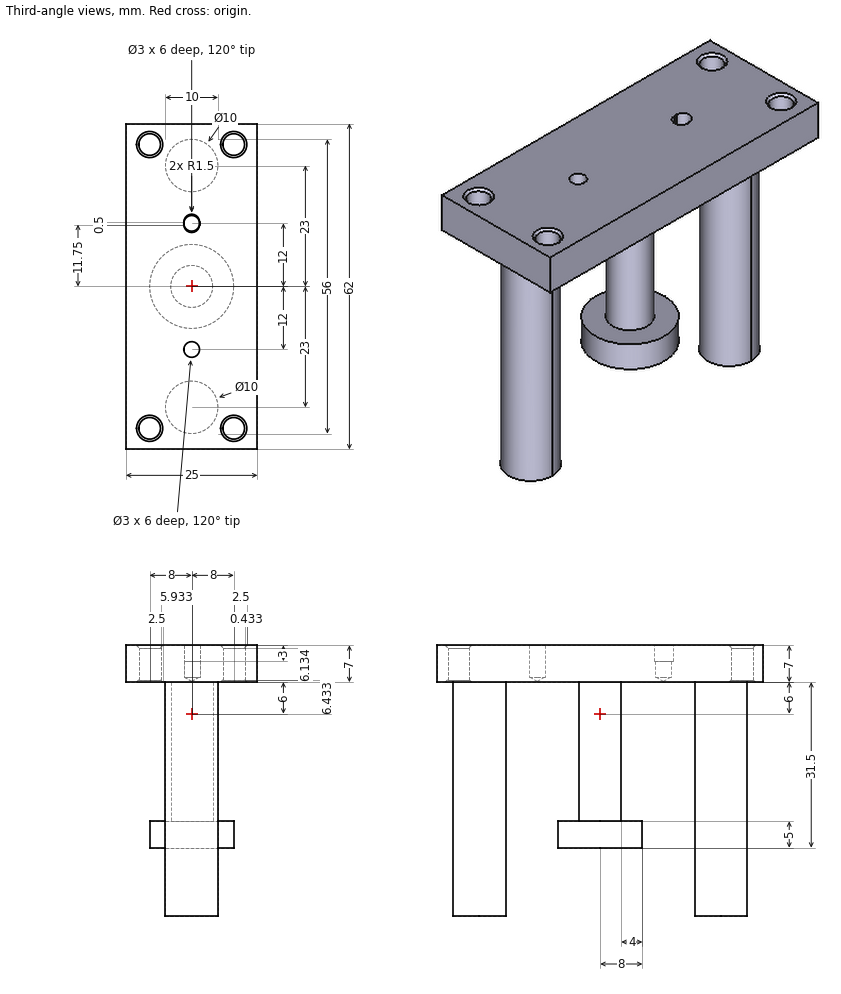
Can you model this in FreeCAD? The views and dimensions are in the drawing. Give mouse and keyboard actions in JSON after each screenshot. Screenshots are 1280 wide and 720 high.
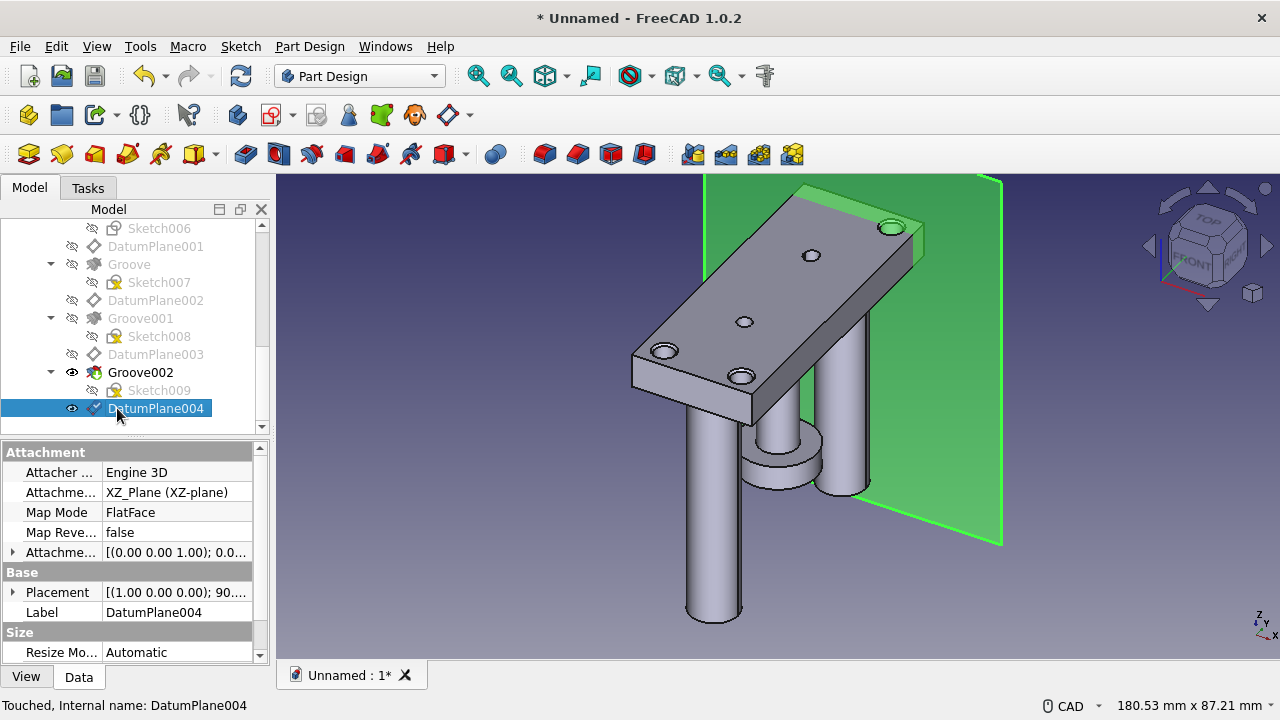
{"action": "left_click", "coordinate": [270, 116]}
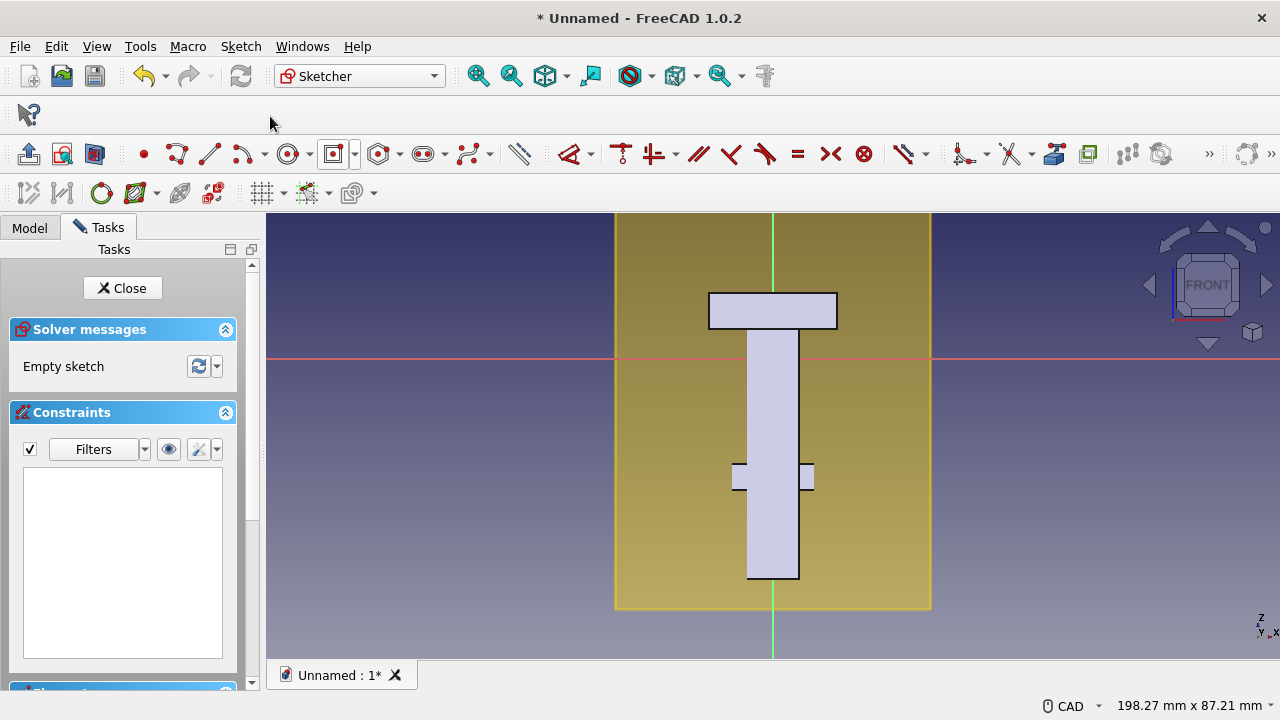
{"action": "left_click", "coordinate": [95, 154]}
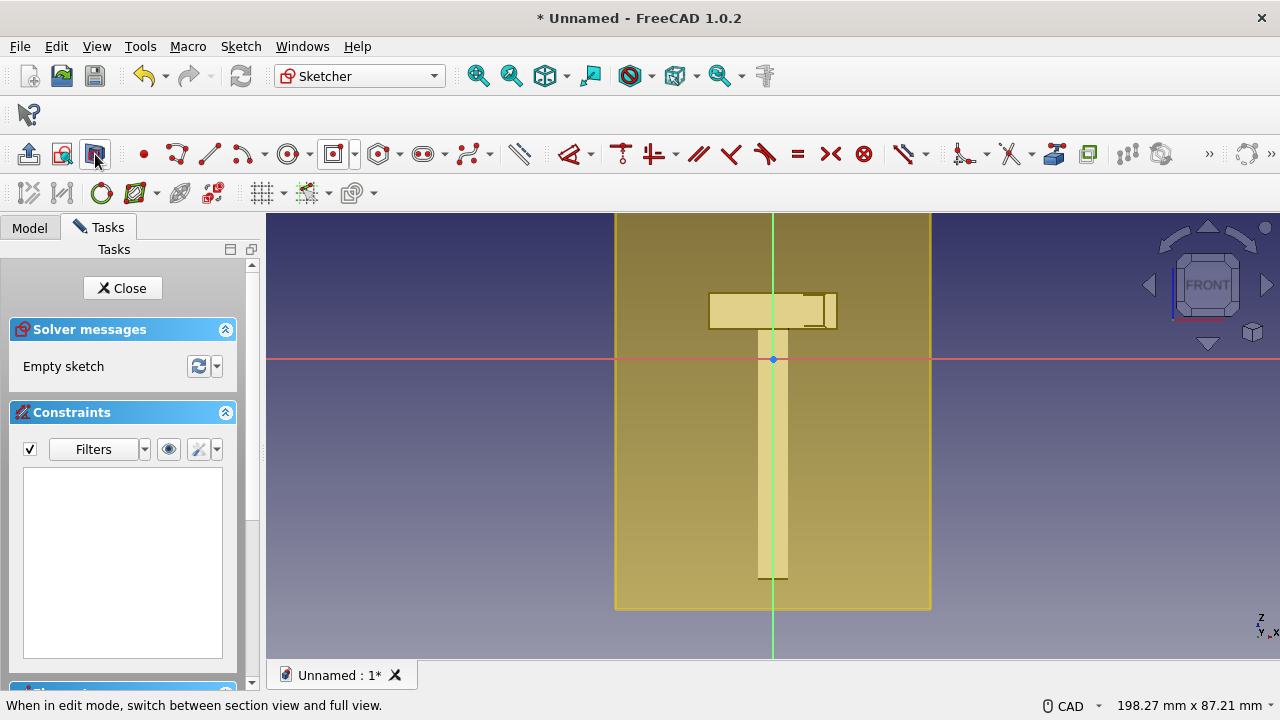
{"action": "scroll", "coordinate": [768, 290], "scroll_direction": "up", "scroll_amount": 7}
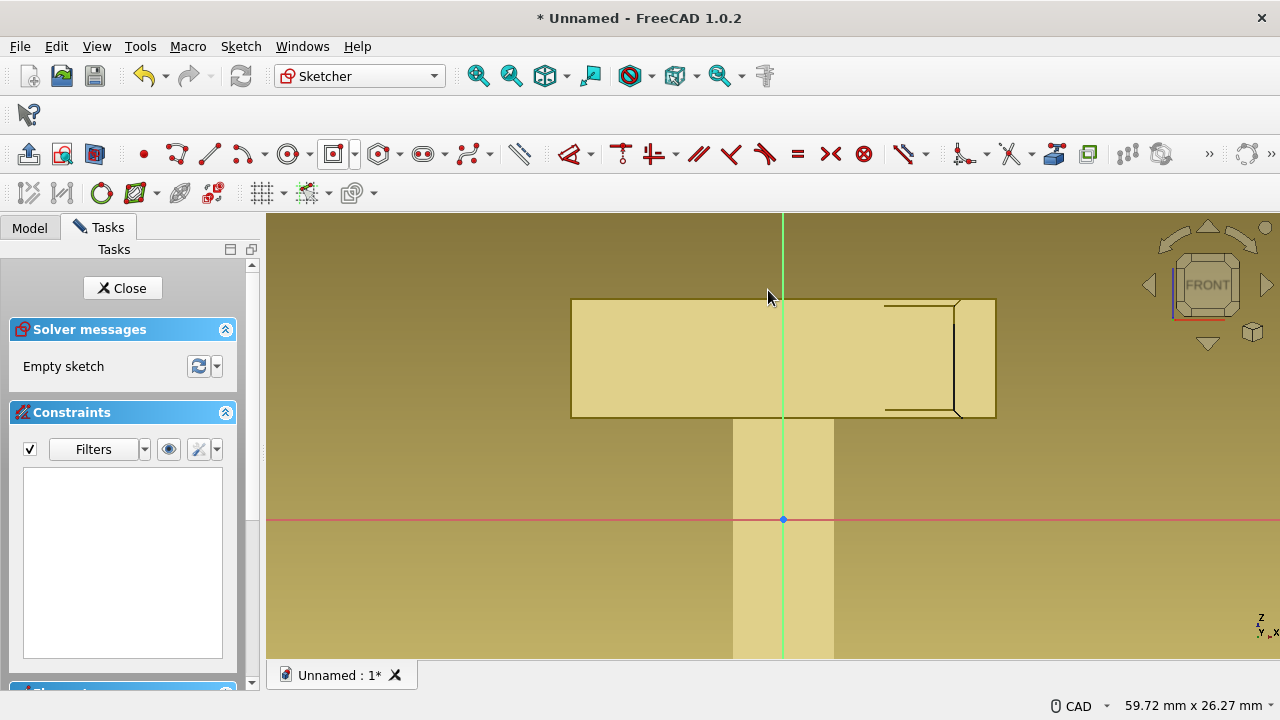
{"action": "left_click", "coordinate": [177, 154]}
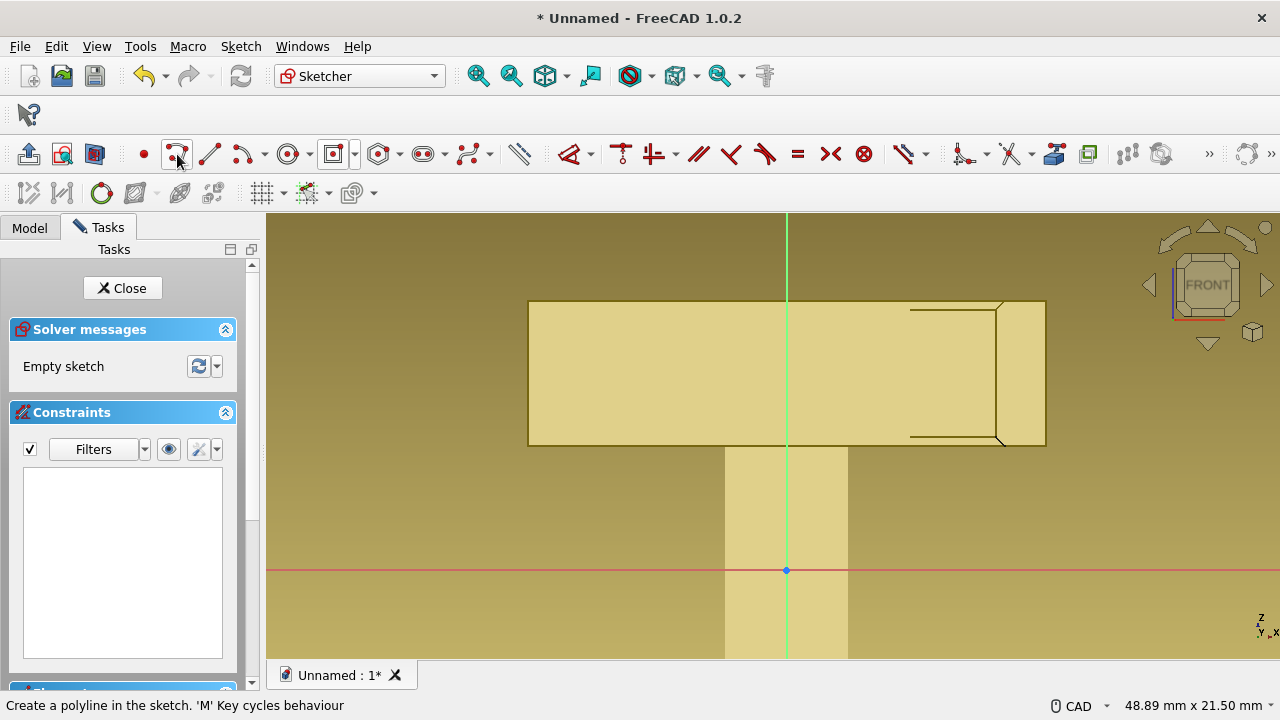
{"action": "left_click", "coordinate": [673, 446]}
{"action": "left_click", "coordinate": [621, 446]}
{"action": "left_click", "coordinate": [621, 301]}
{"action": "left_click", "coordinate": [673, 301]}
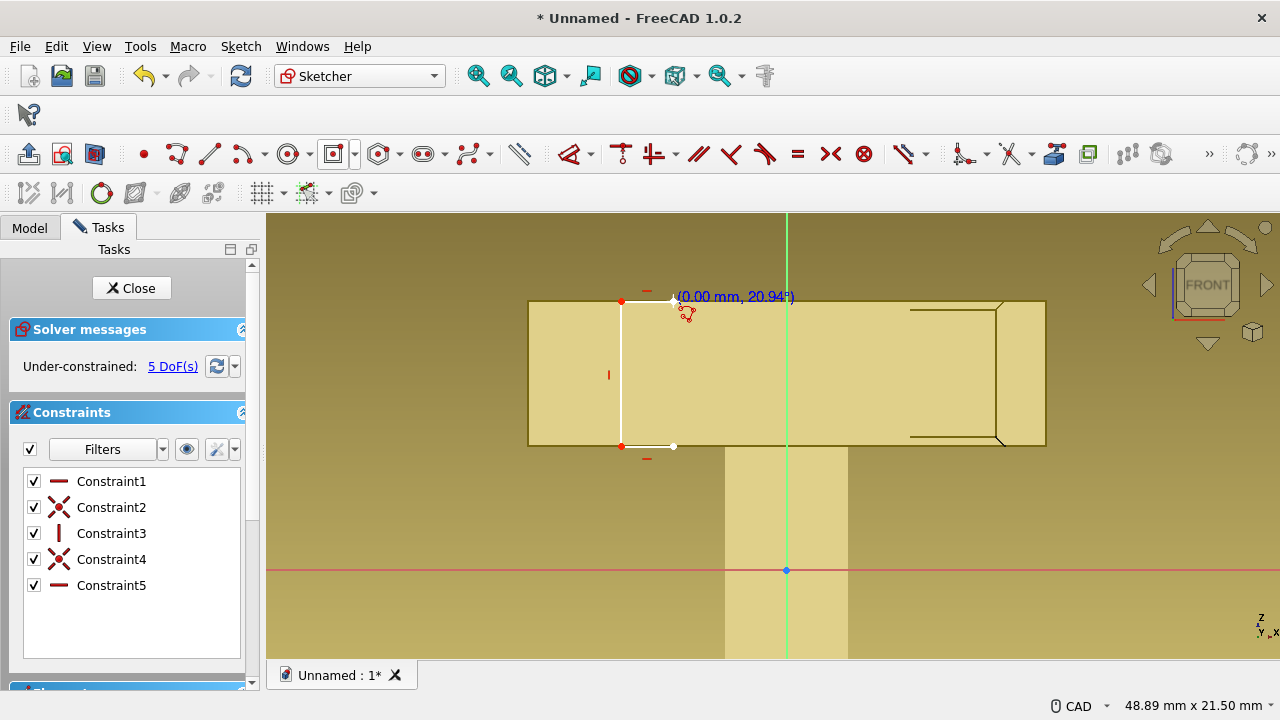
{"action": "scroll", "coordinate": [664, 310], "scroll_direction": "up", "scroll_amount": 3}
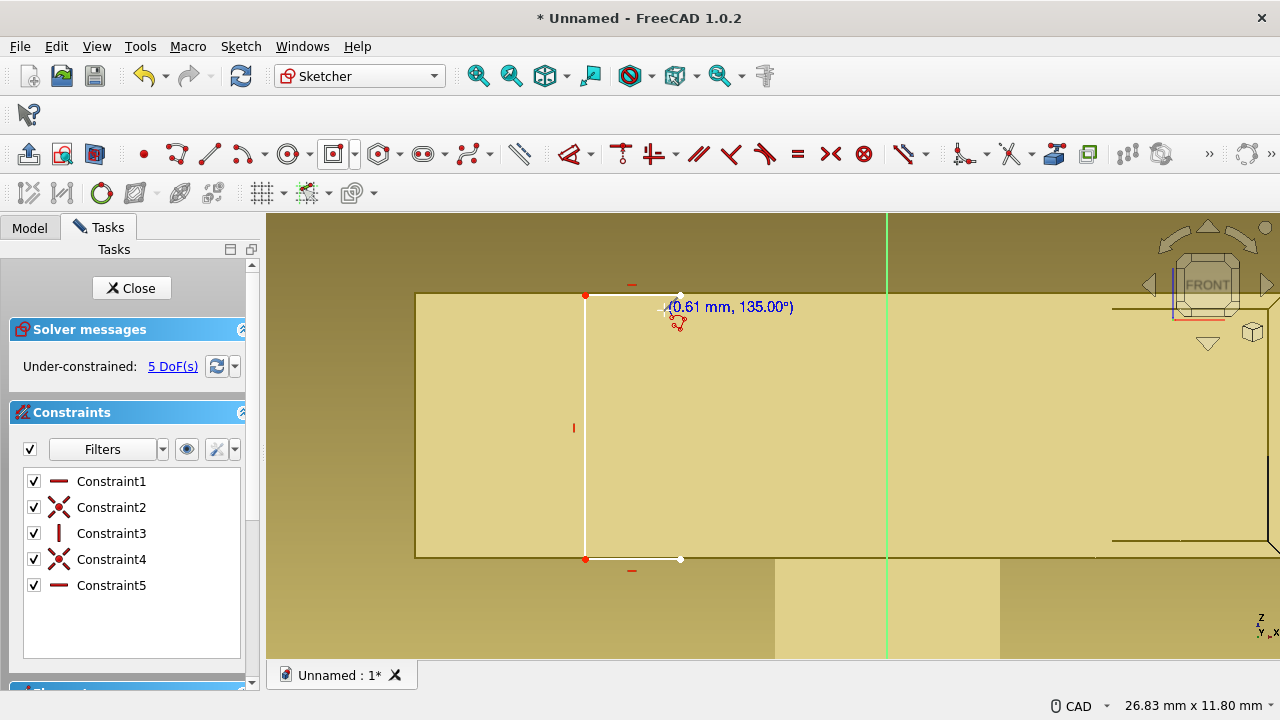
{"action": "left_click", "coordinate": [663, 309]}
{"action": "left_click", "coordinate": [663, 541]}
{"action": "left_click", "coordinate": [680, 559]}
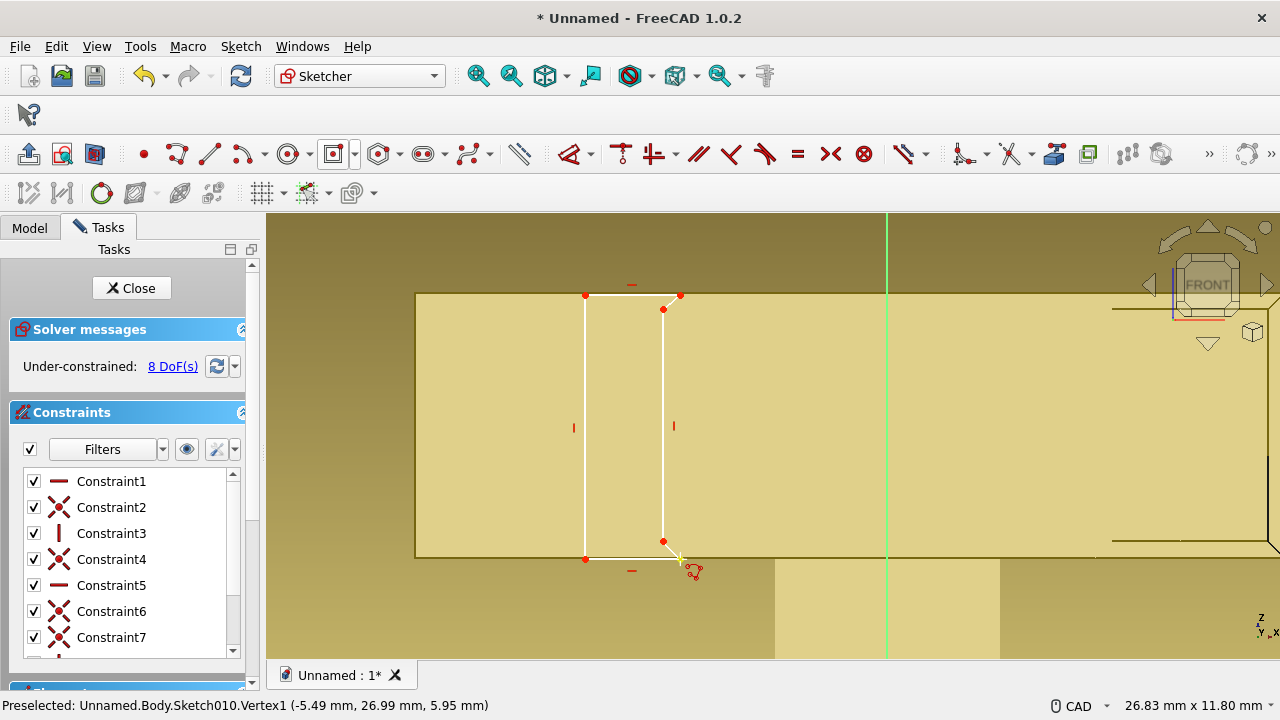
{"action": "left_click", "coordinate": [210, 154]}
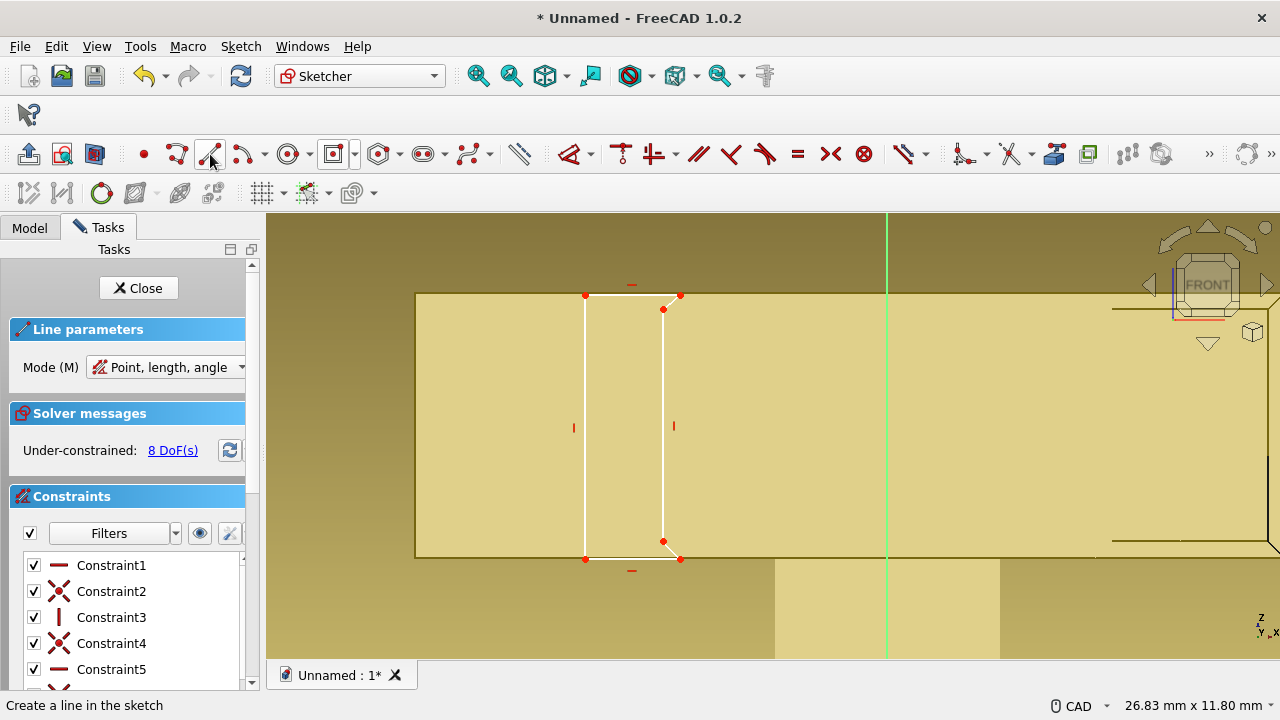
{"action": "left_click", "coordinate": [585, 584]}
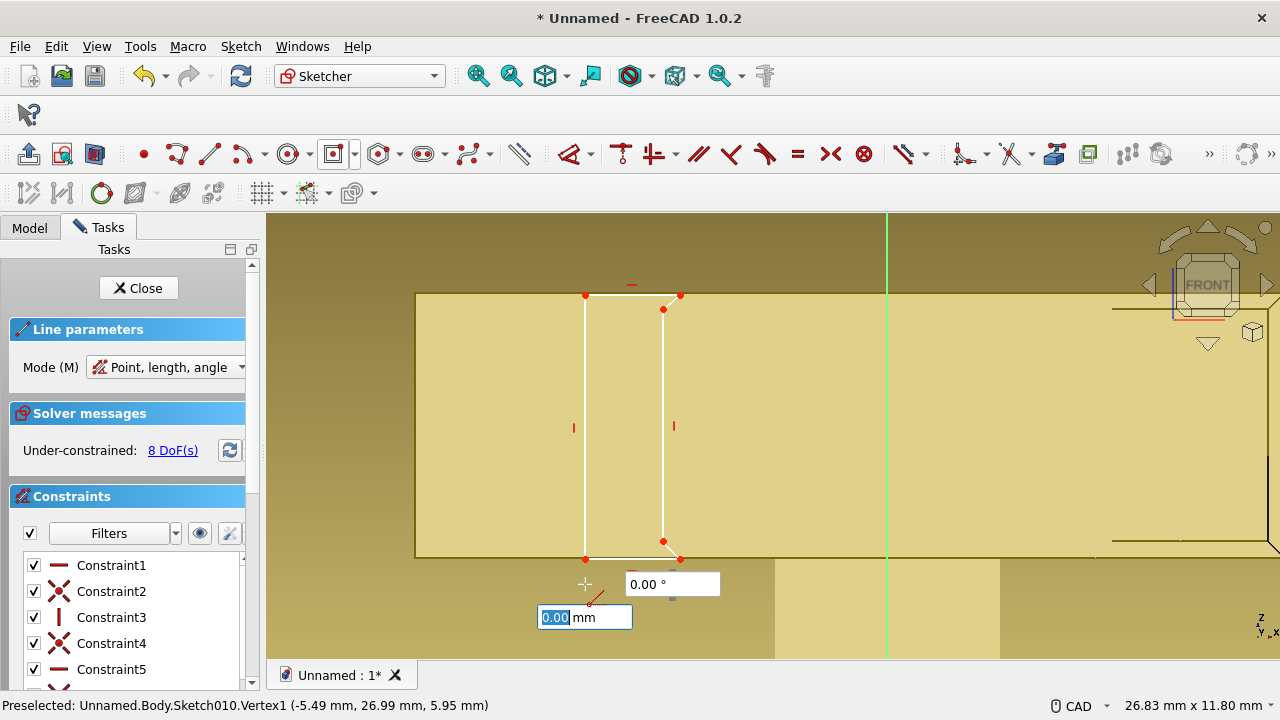
{"action": "scroll", "coordinate": [666, 311], "scroll_direction": "down", "scroll_amount": 3}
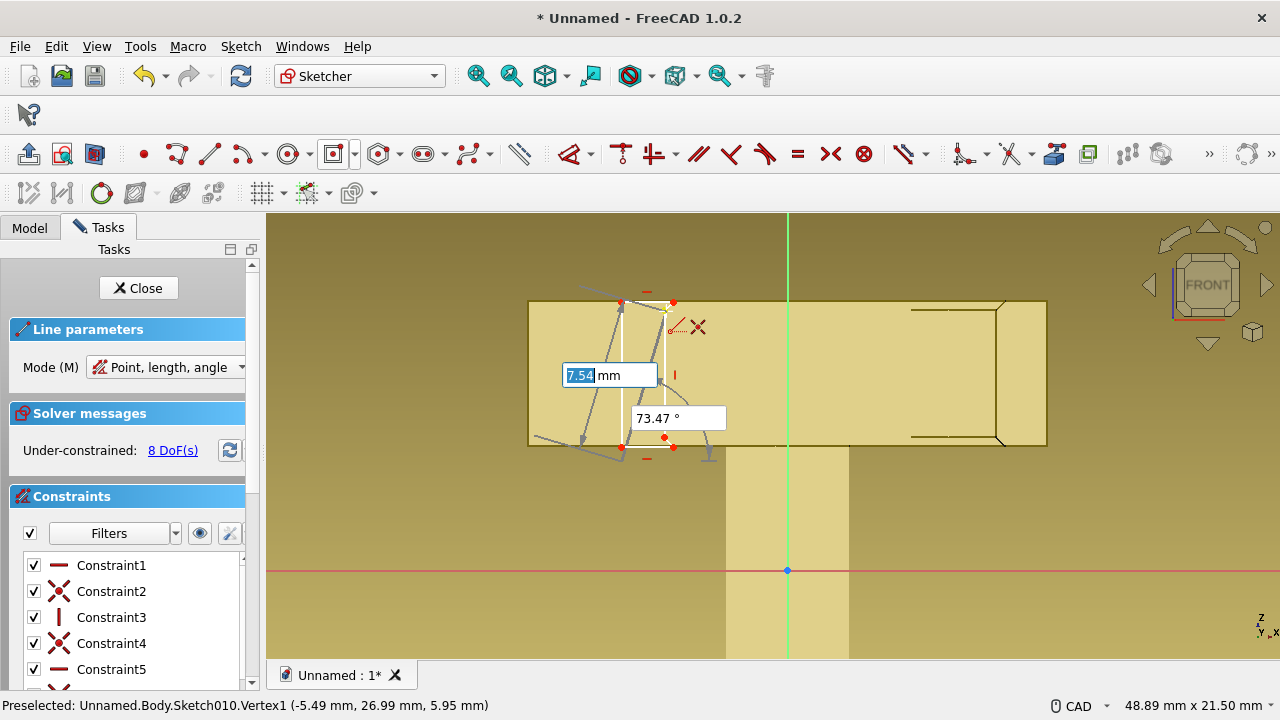
{"action": "left_click", "coordinate": [622, 505]}
{"action": "key", "text": "Escape"}